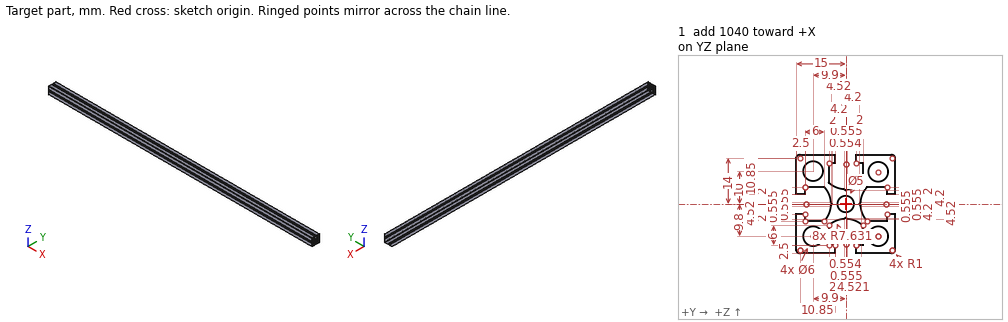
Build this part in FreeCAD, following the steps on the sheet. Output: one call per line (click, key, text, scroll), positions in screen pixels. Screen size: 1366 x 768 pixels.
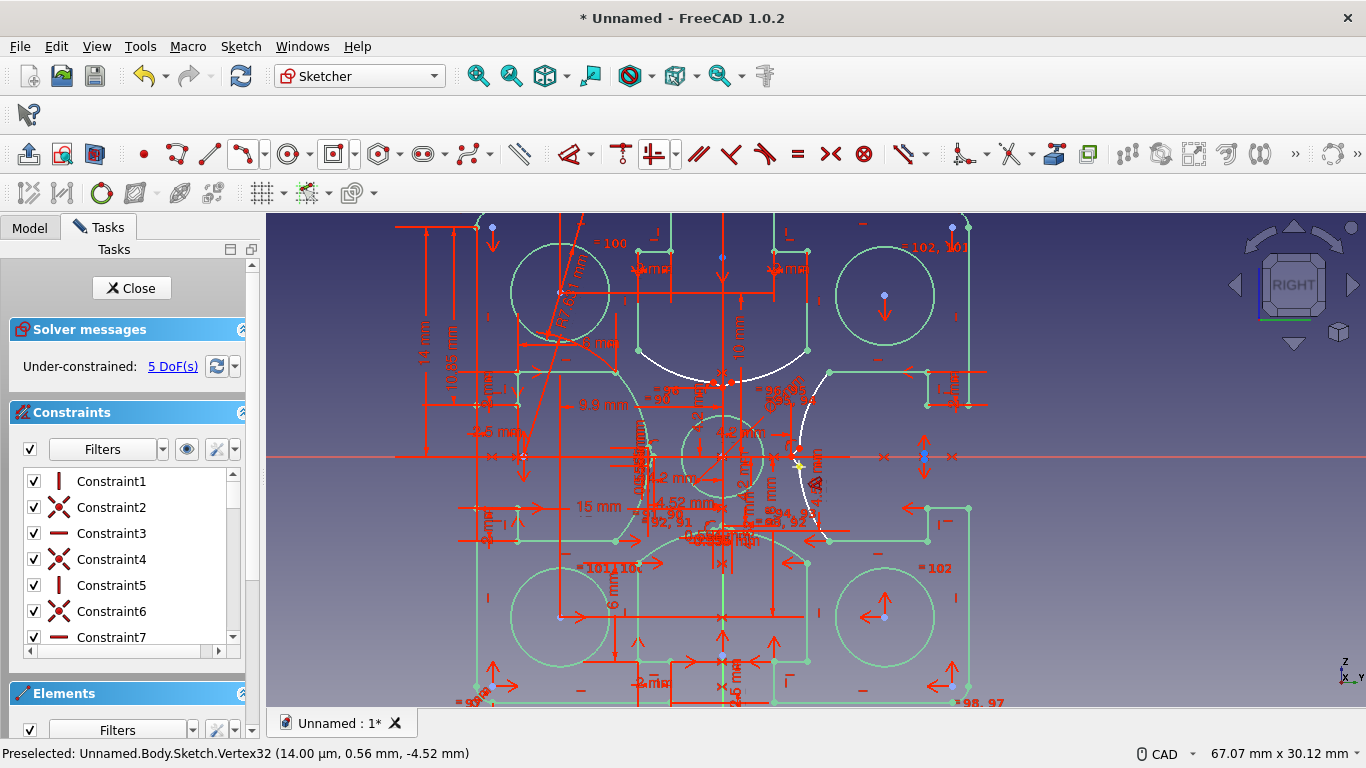
click(799, 466)
click(761, 572)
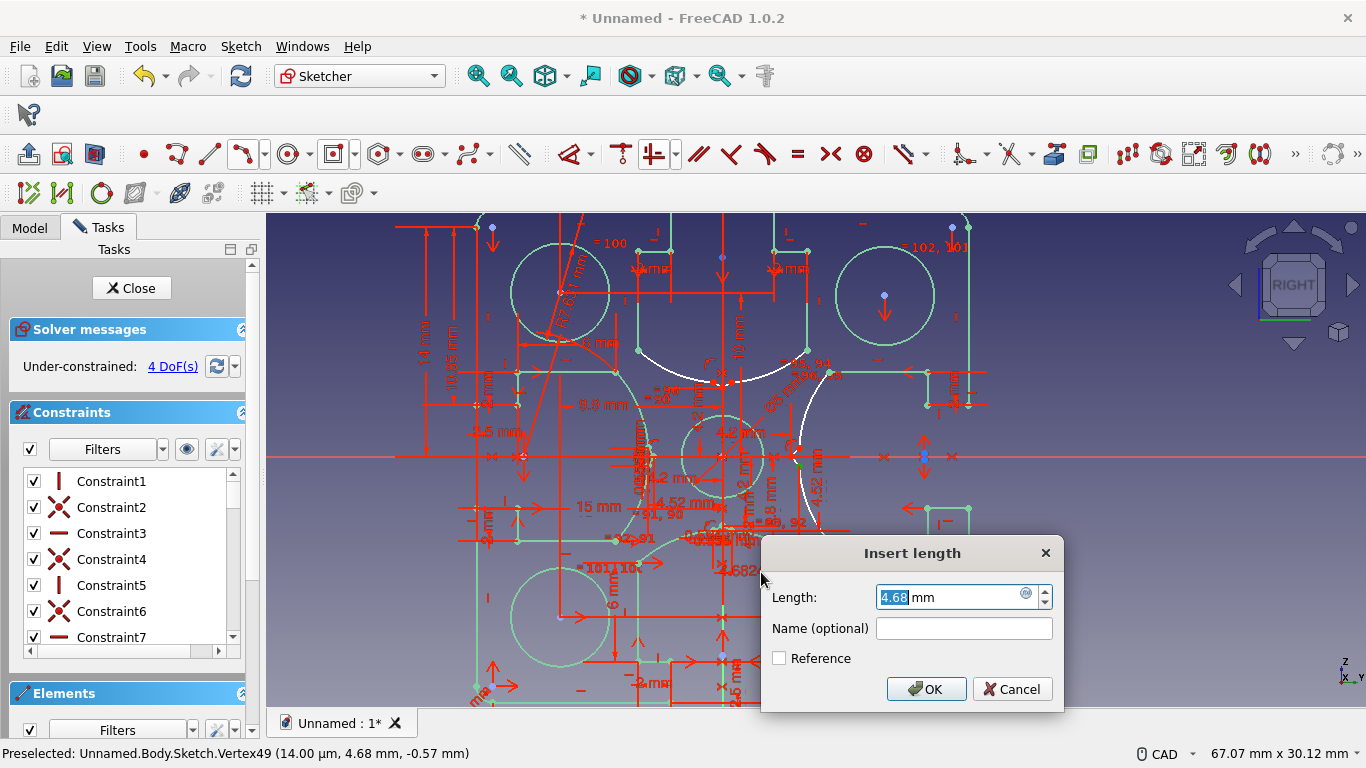
text(4.521)
key(Return)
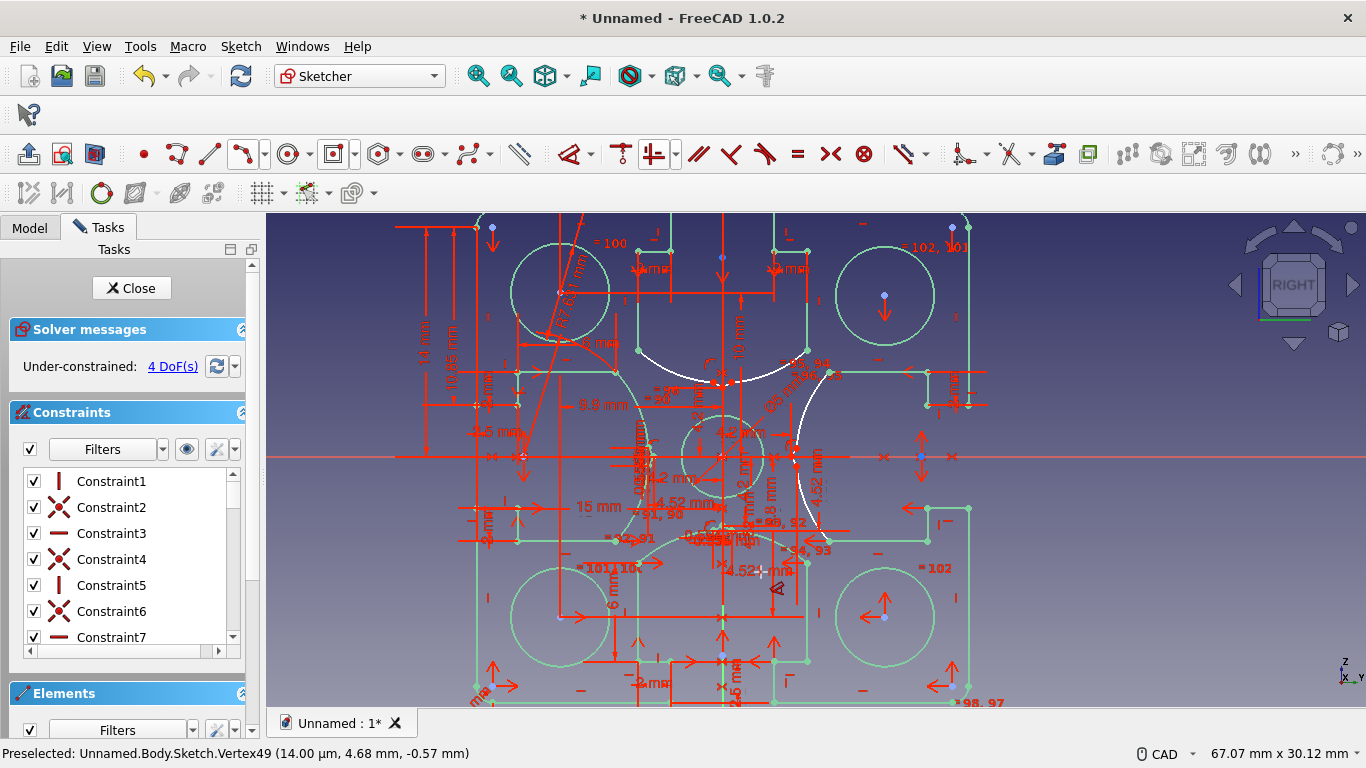
scroll(797, 466, up, 8)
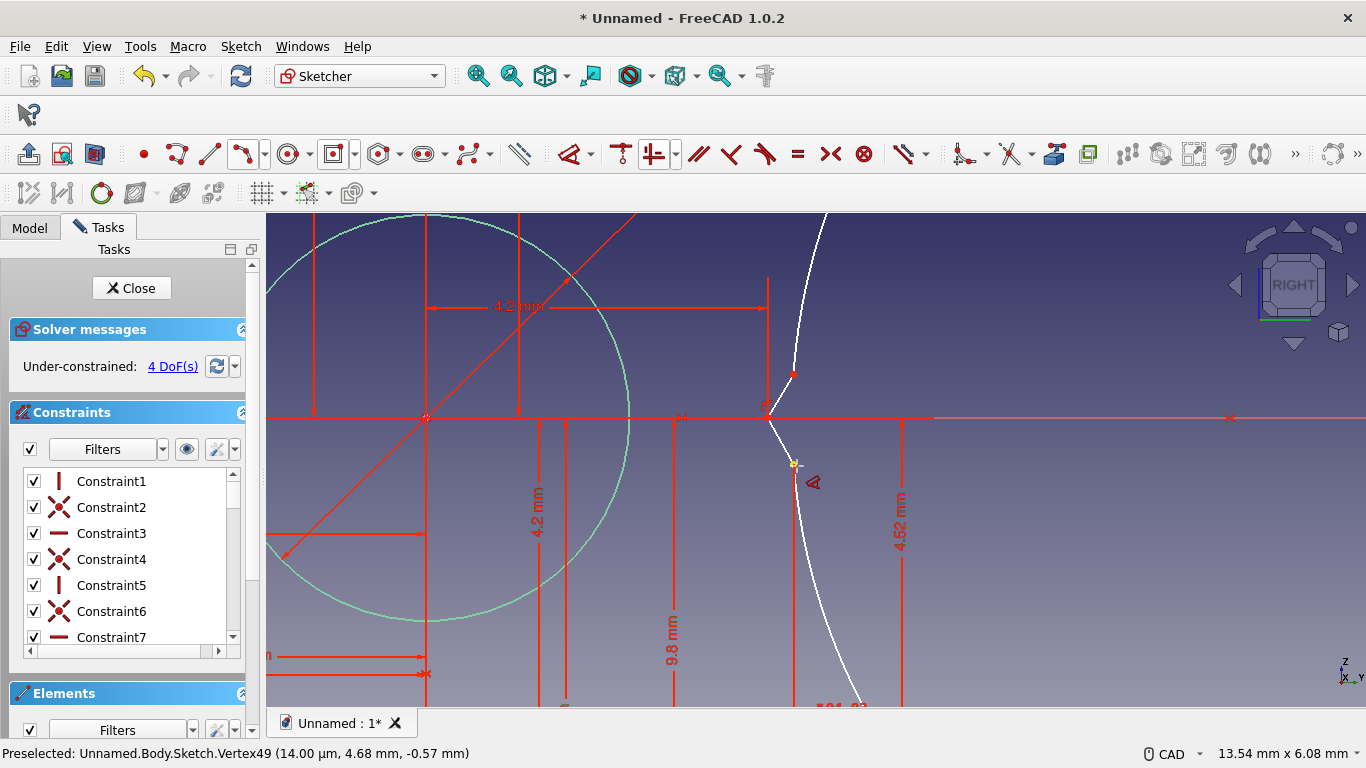
click(794, 465)
click(828, 441)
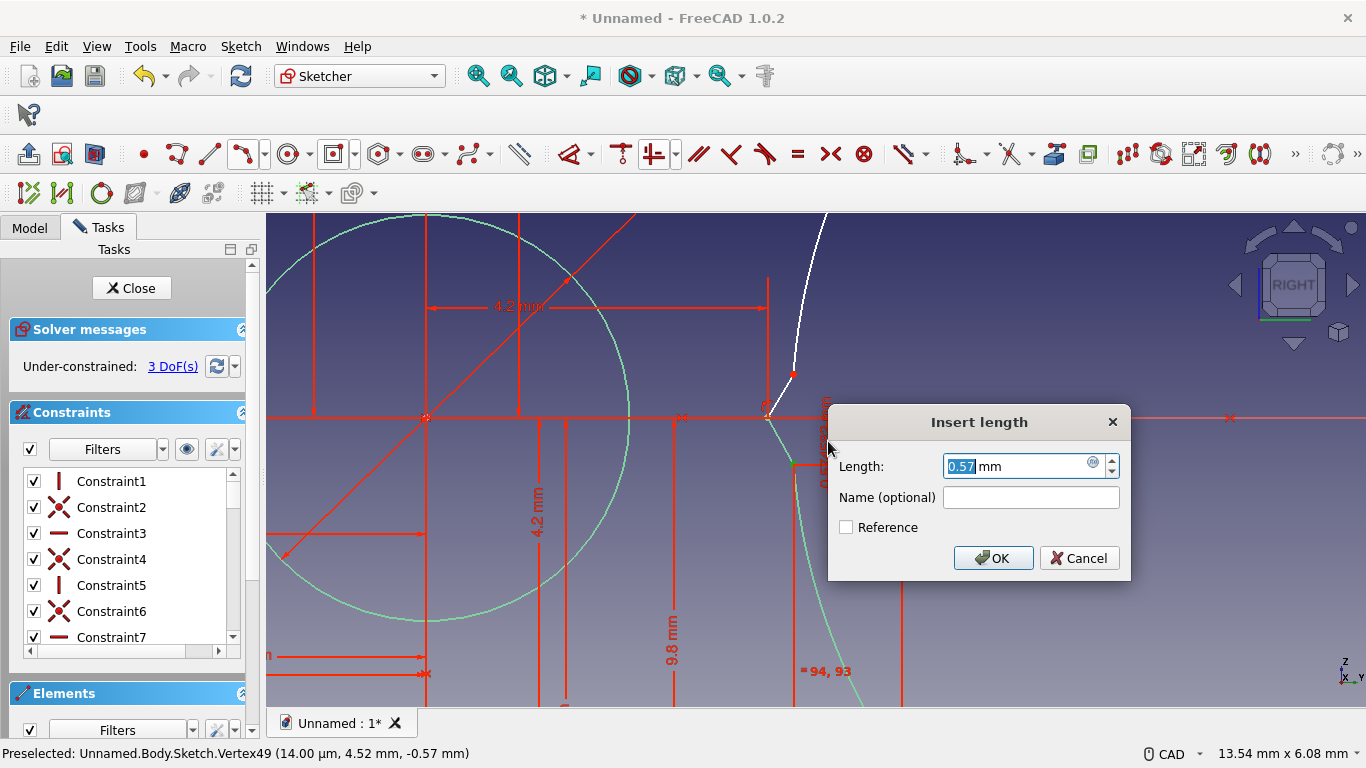
text(0.555)
key(Return)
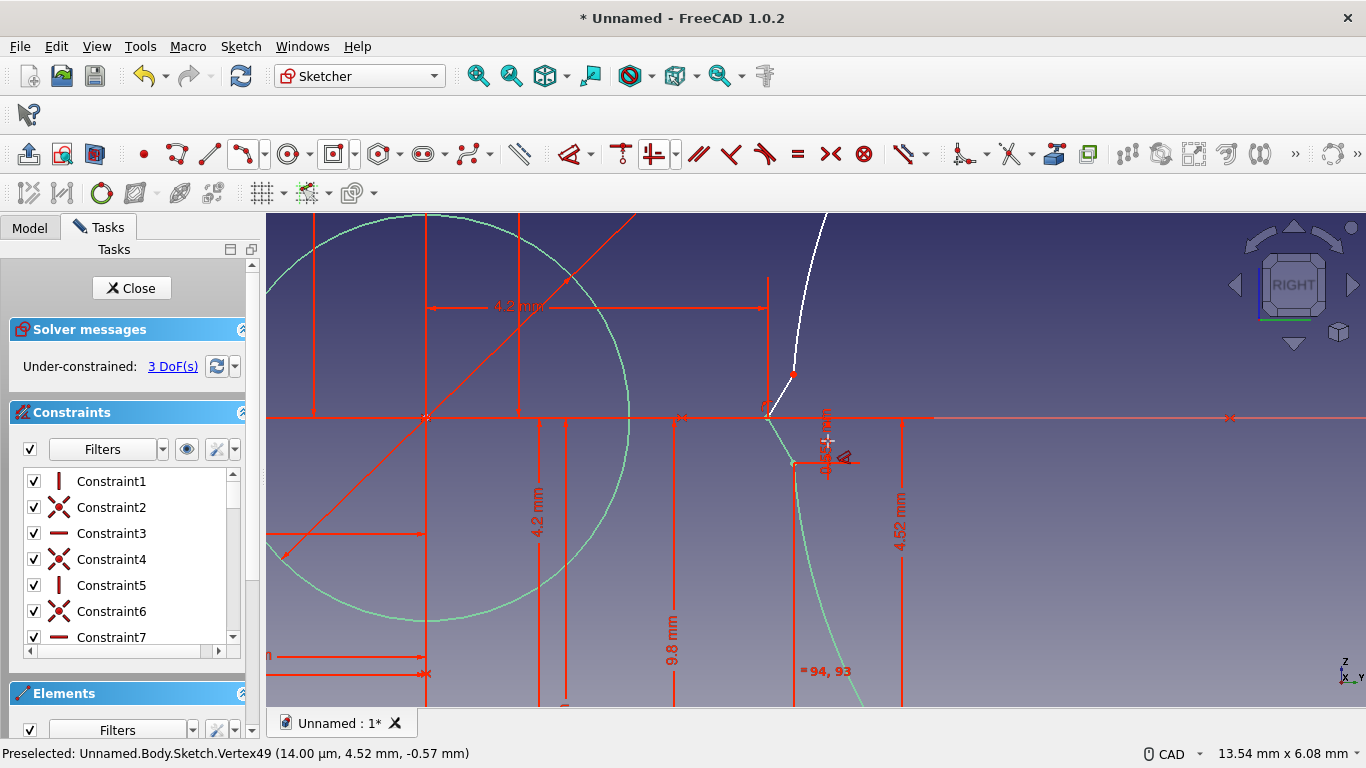
click(794, 375)
click(828, 396)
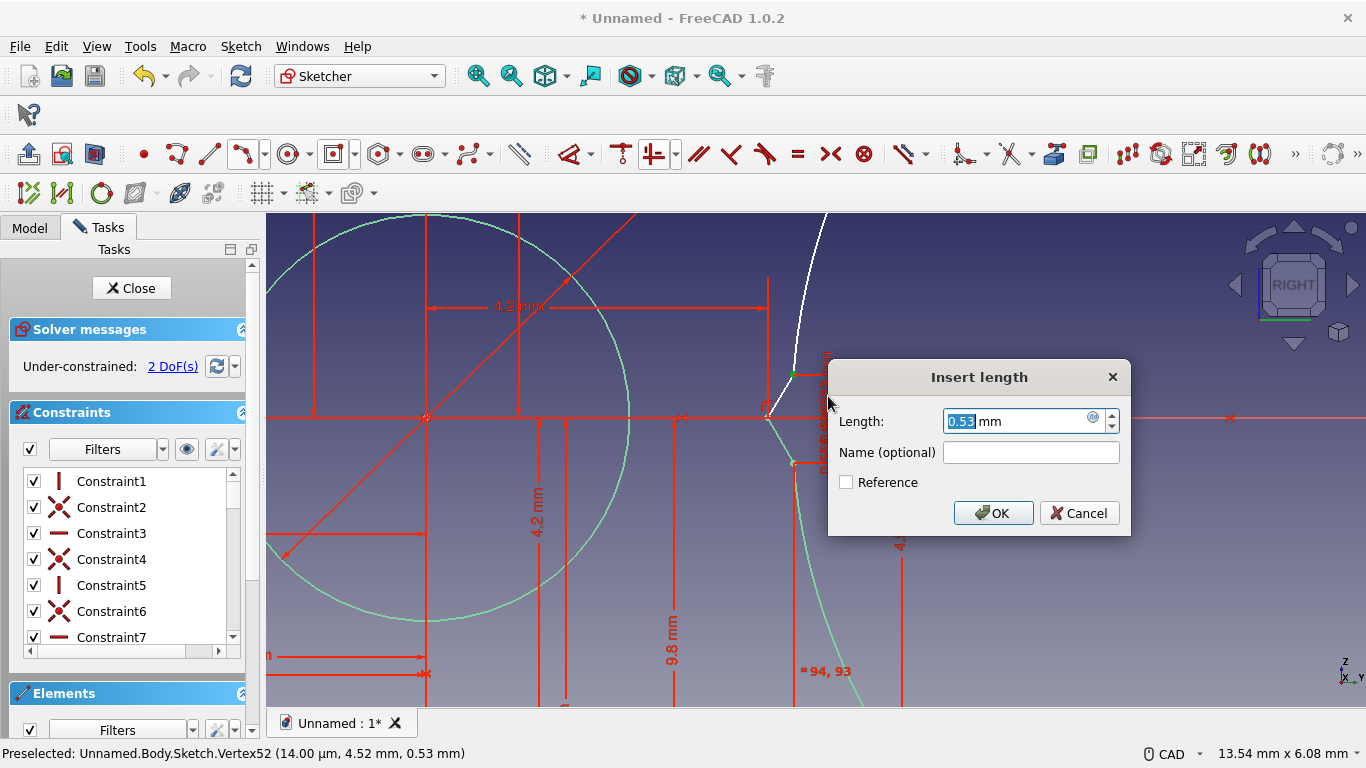
text(0.555)
key(Return)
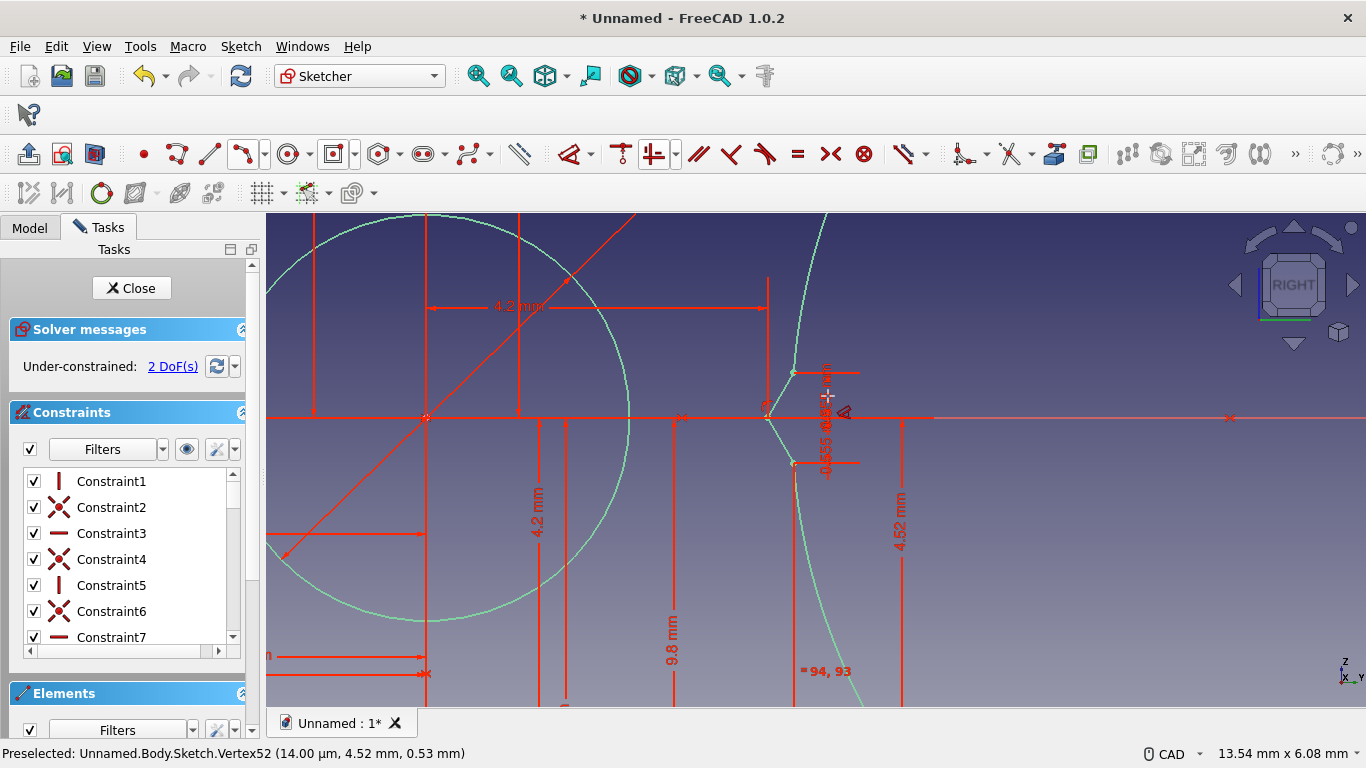
scroll(798, 467, down, 10)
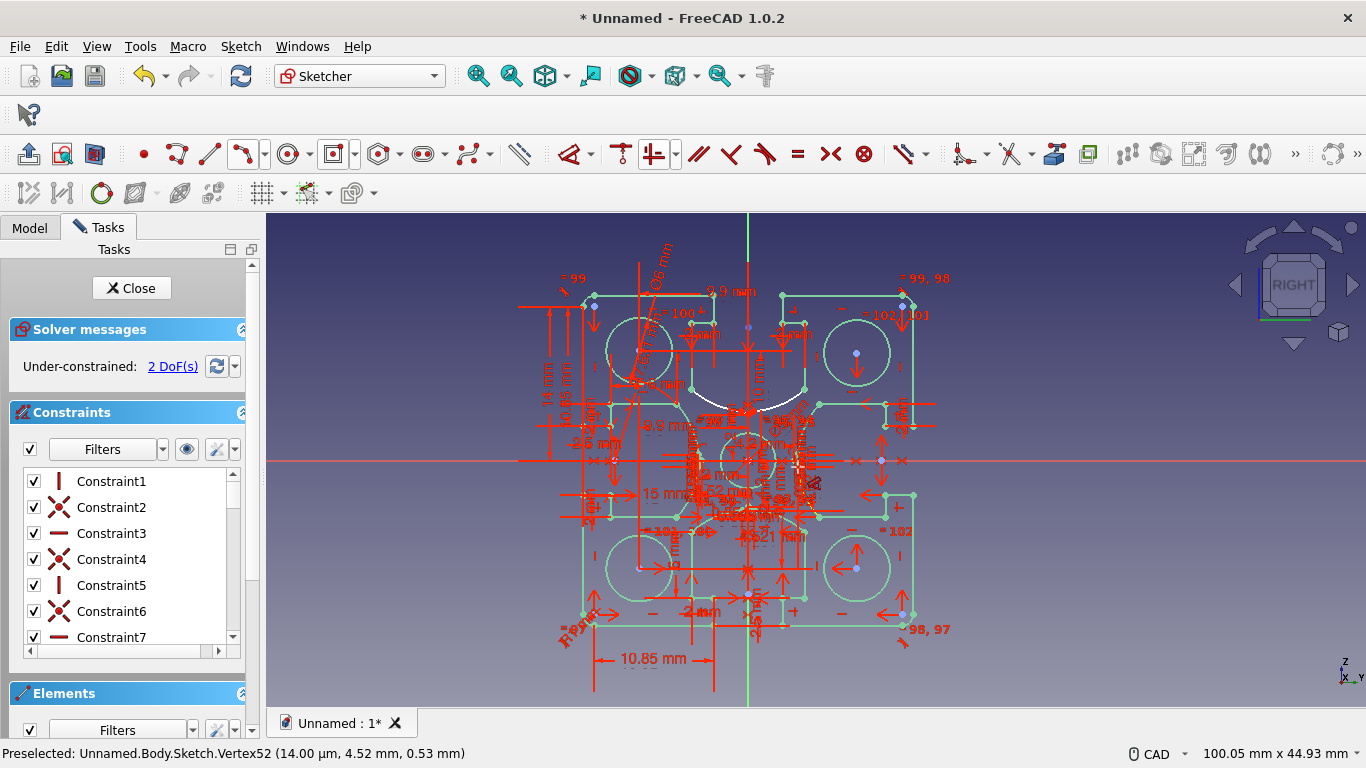
scroll(754, 411, up, 10)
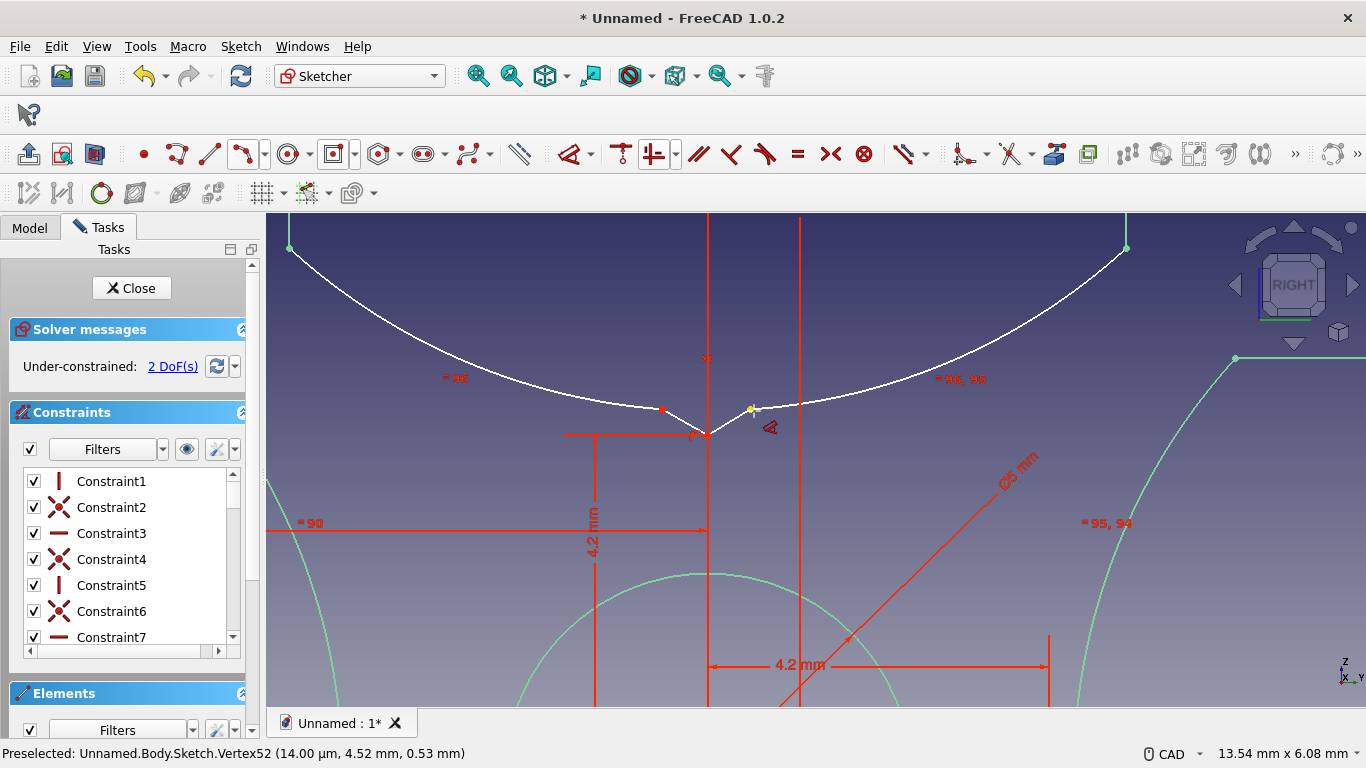
click(750, 409)
click(729, 375)